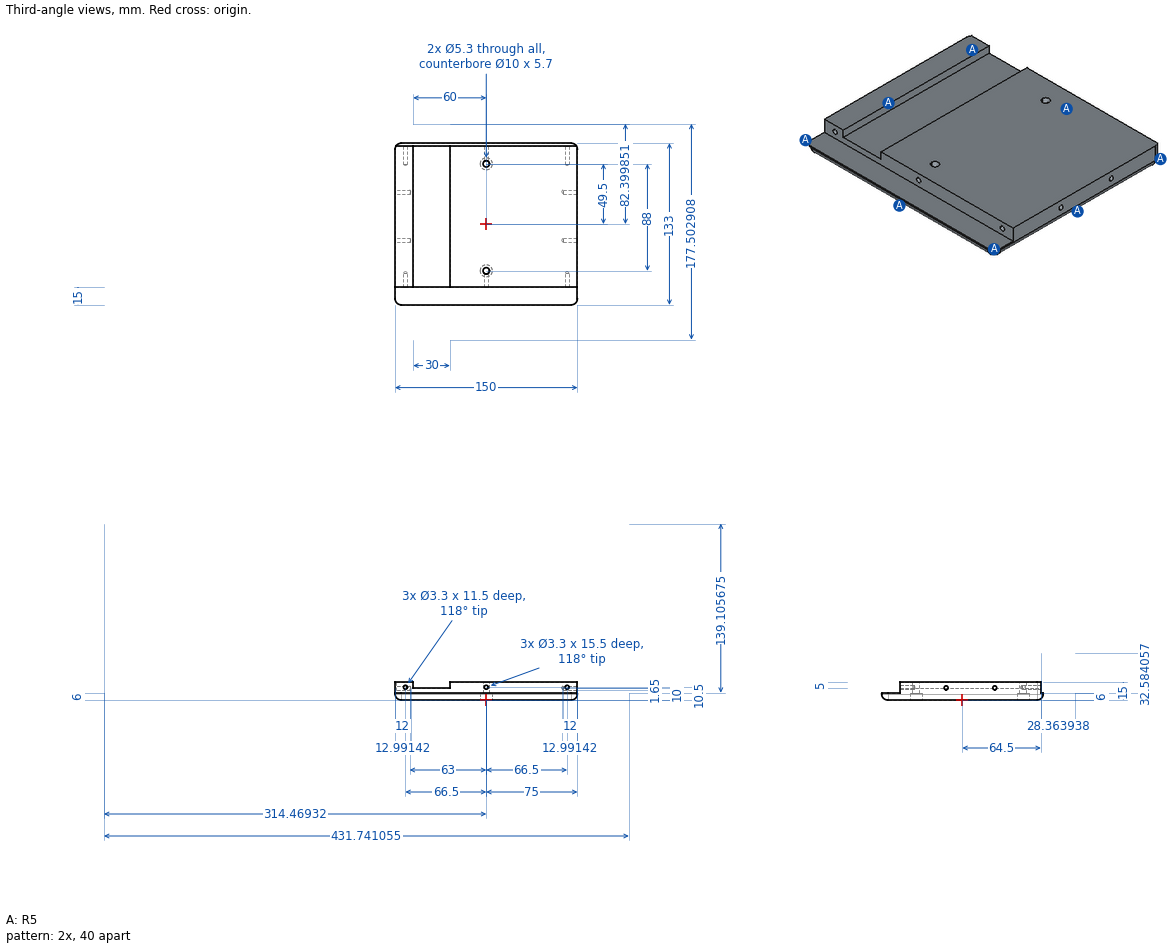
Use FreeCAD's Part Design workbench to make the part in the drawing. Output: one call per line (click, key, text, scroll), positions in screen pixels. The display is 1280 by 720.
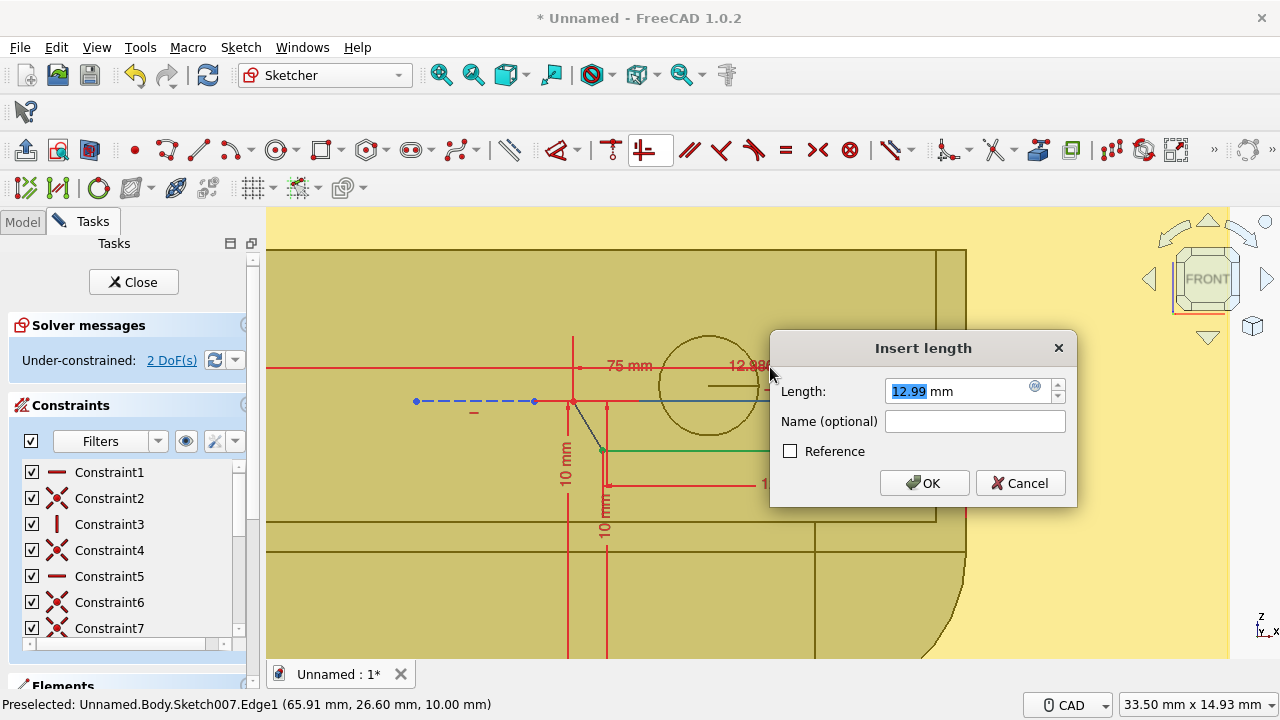
text(12.99142)
key(Return)
key(Escape)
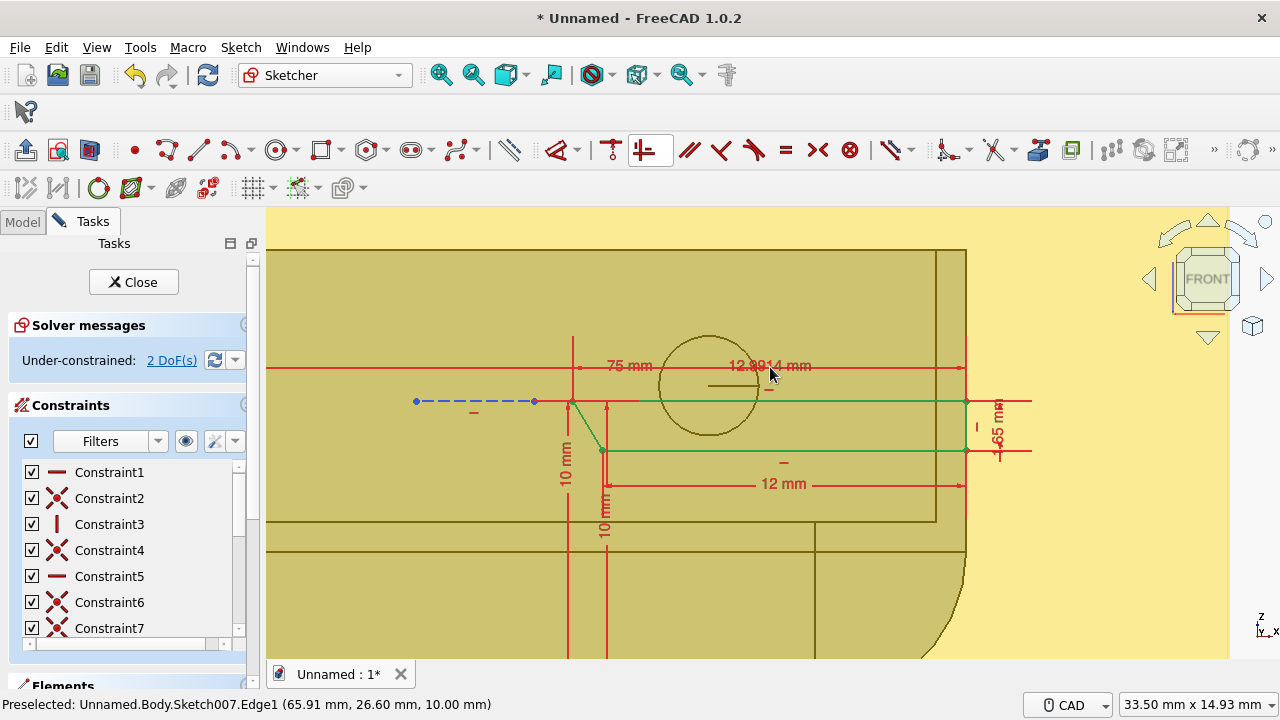
click(134, 282)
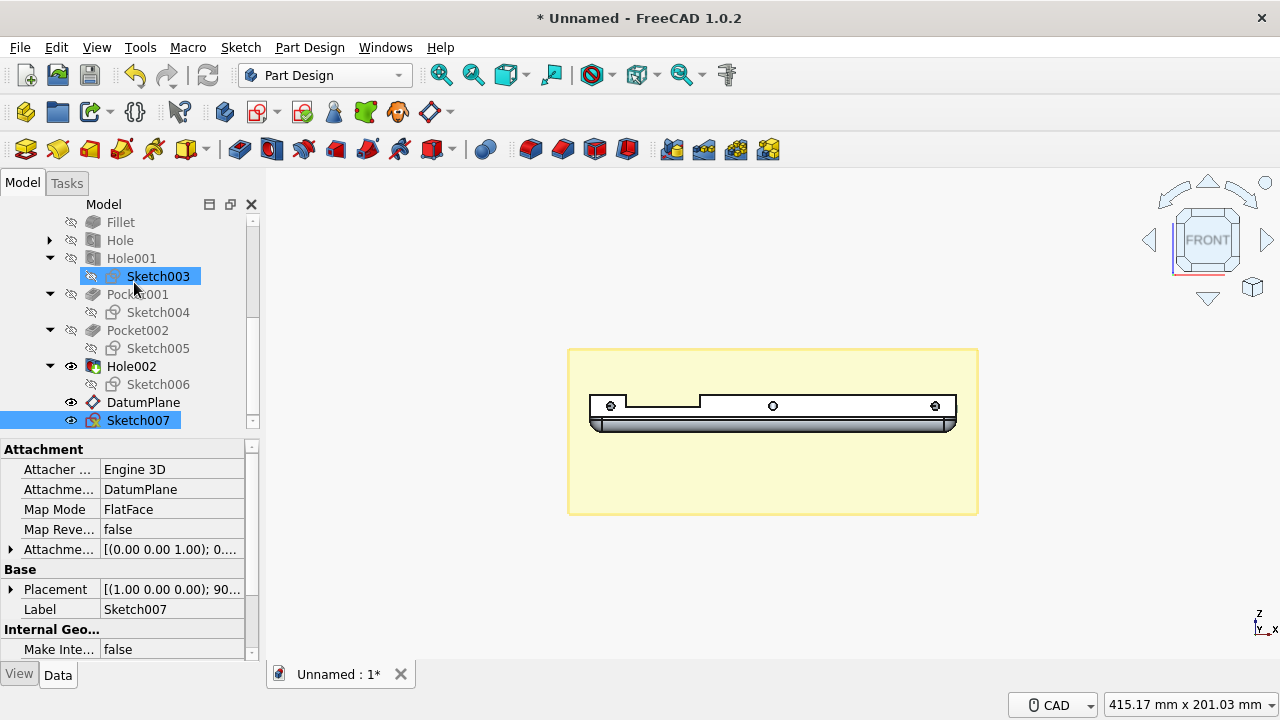
click(304, 150)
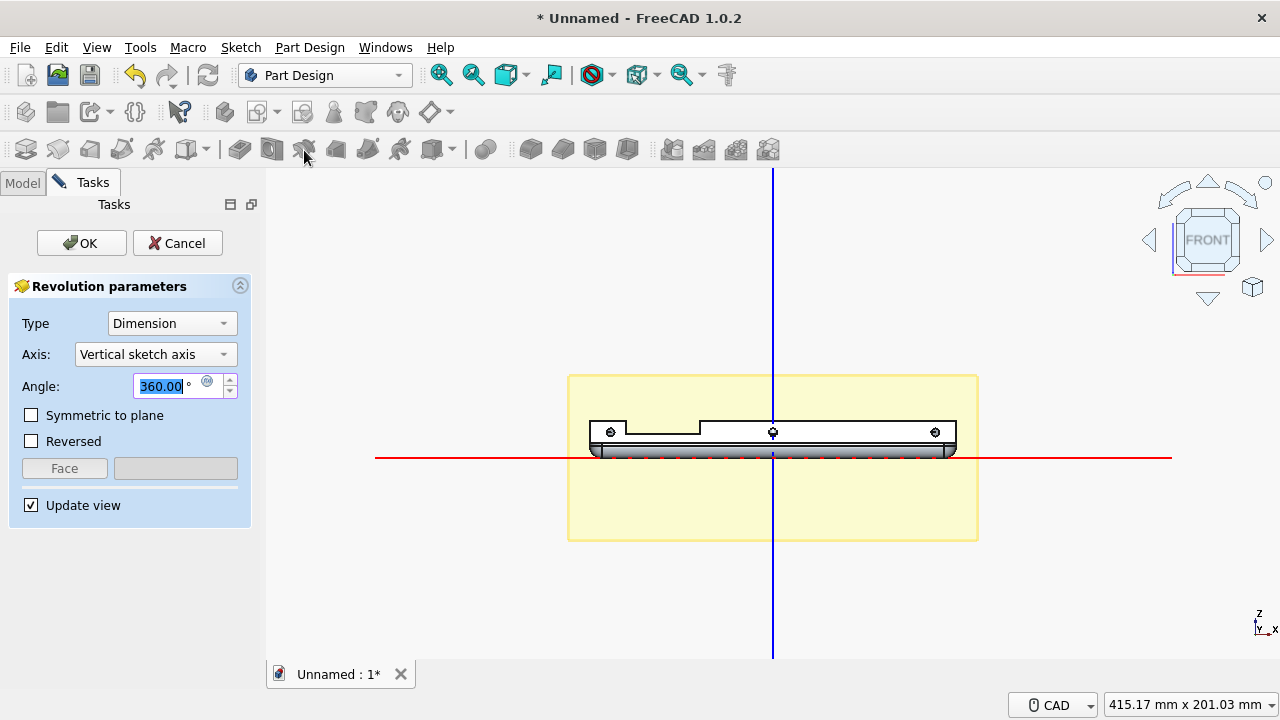
click(156, 354)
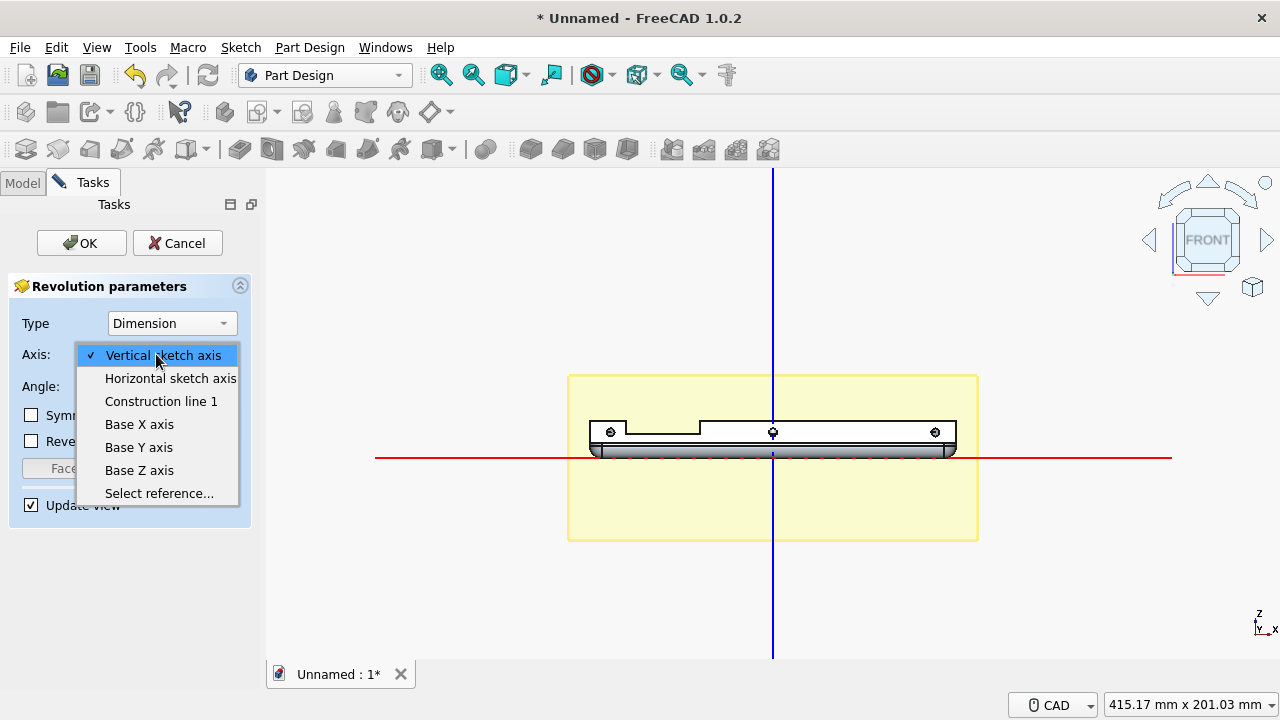
click(156, 402)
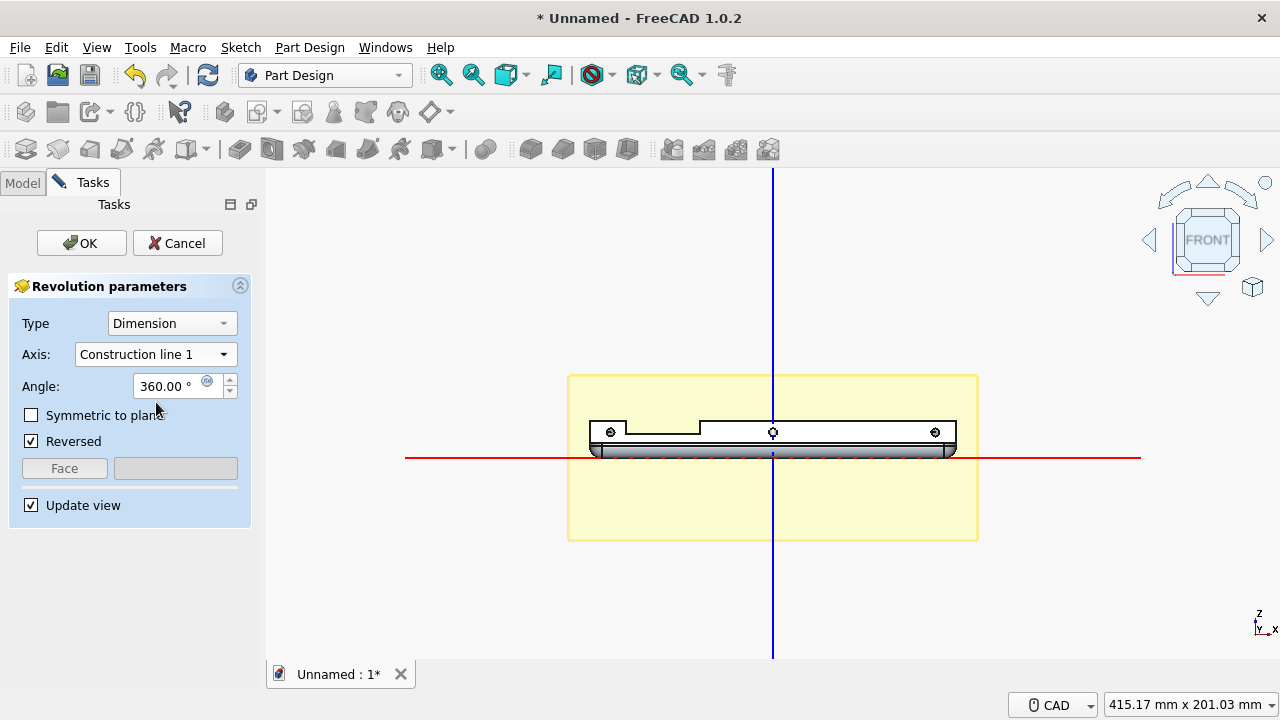
click(82, 243)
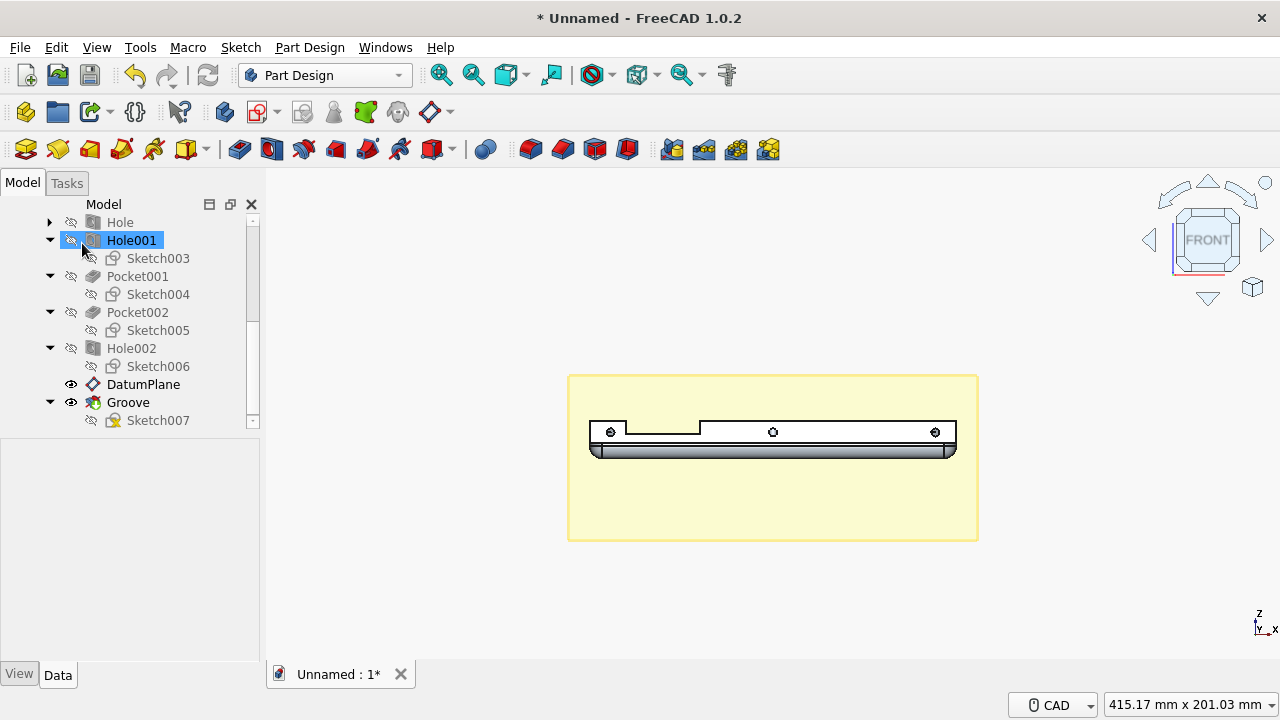
click(116, 384)
key(space)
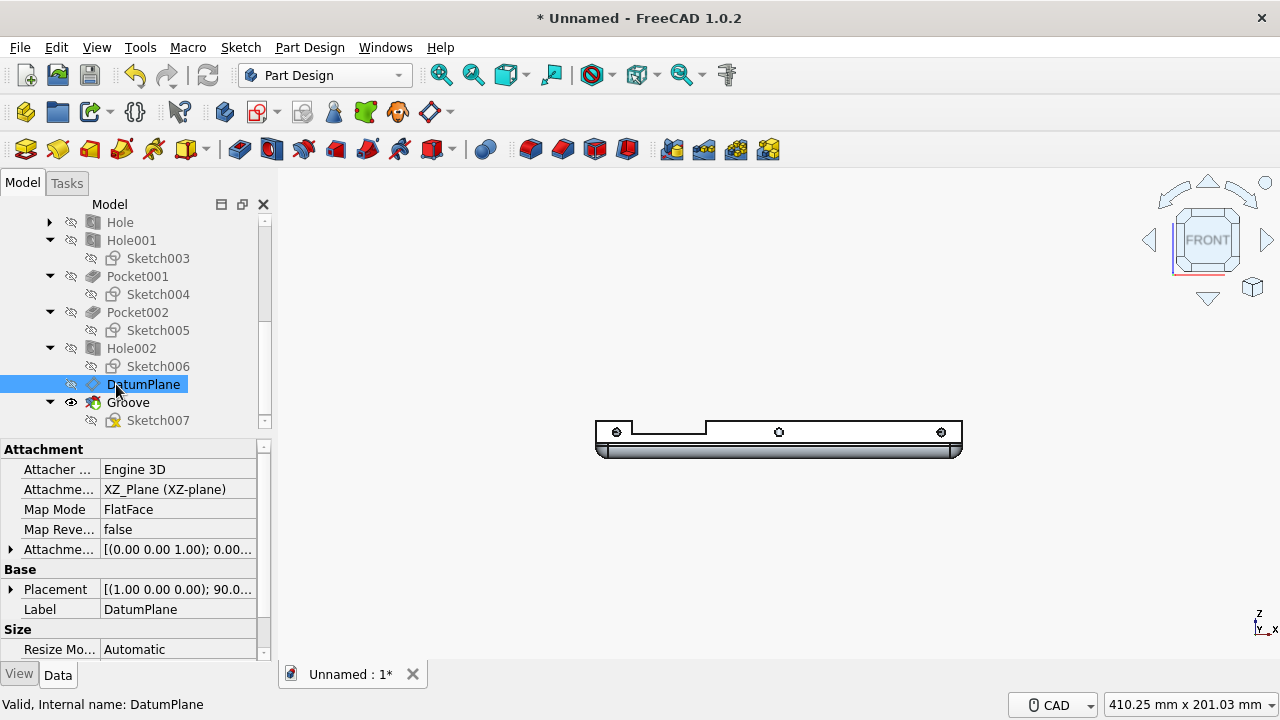
click(442, 76)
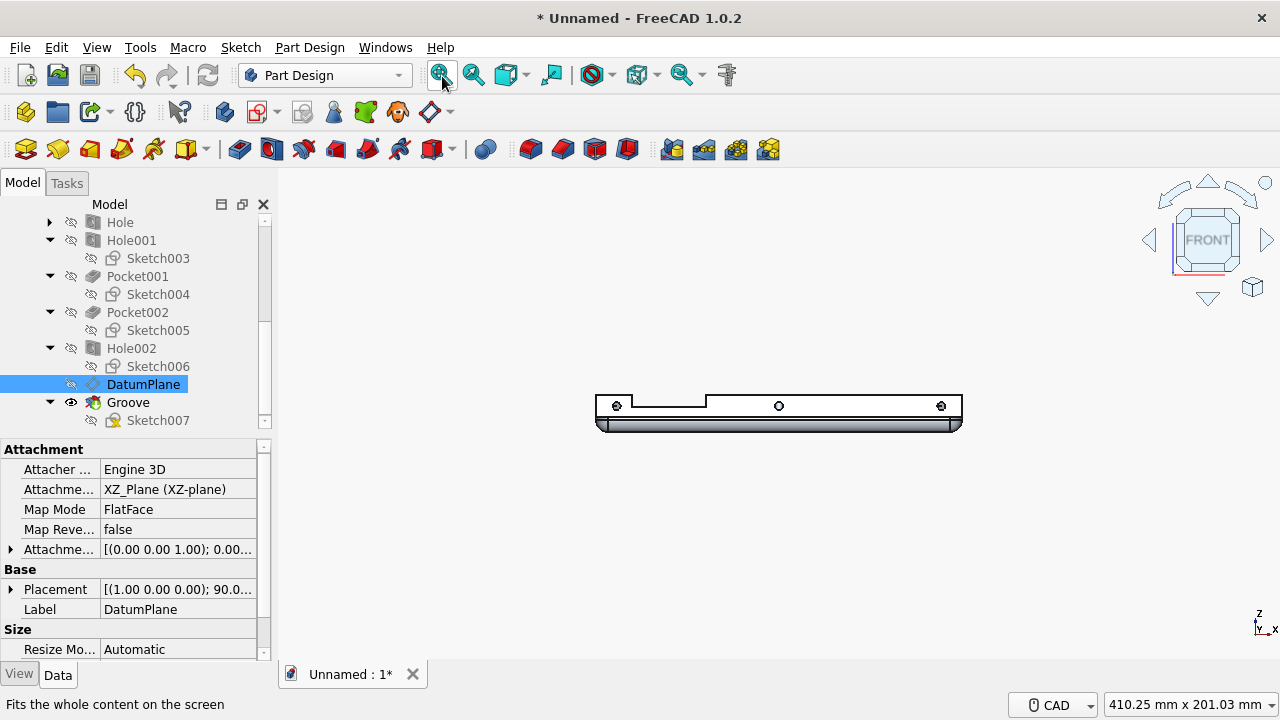
click(116, 402)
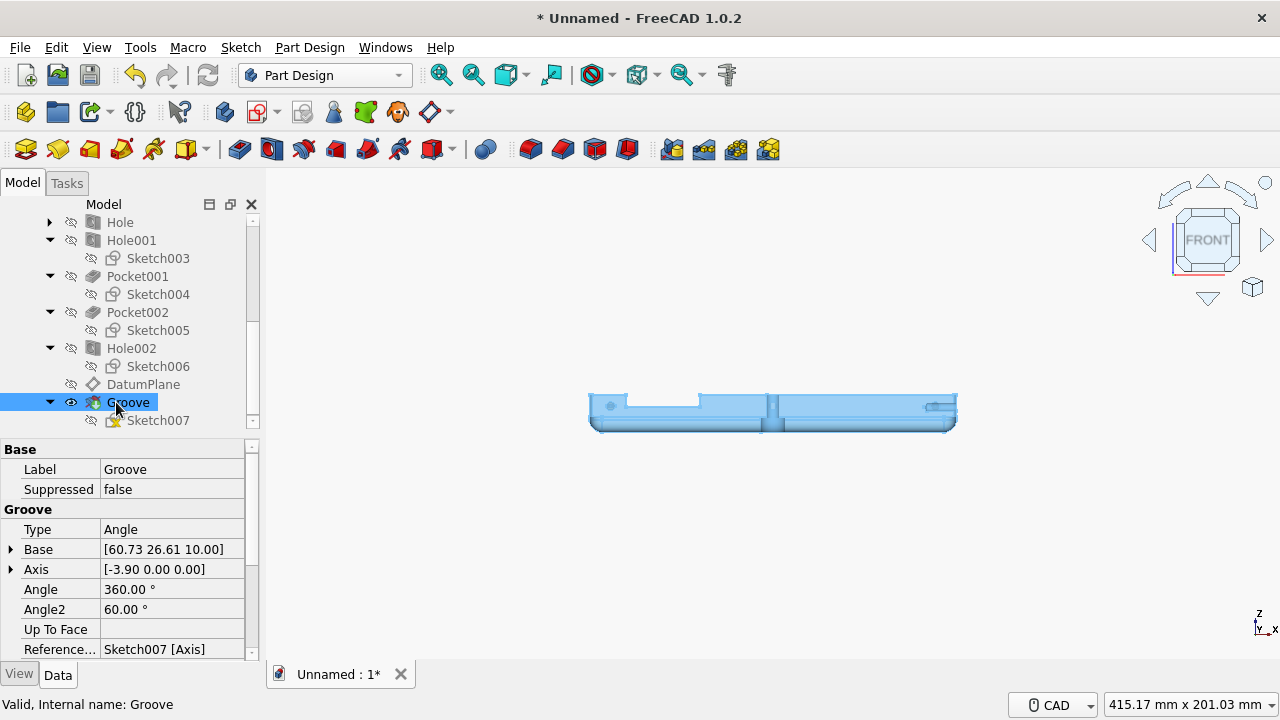
click(704, 150)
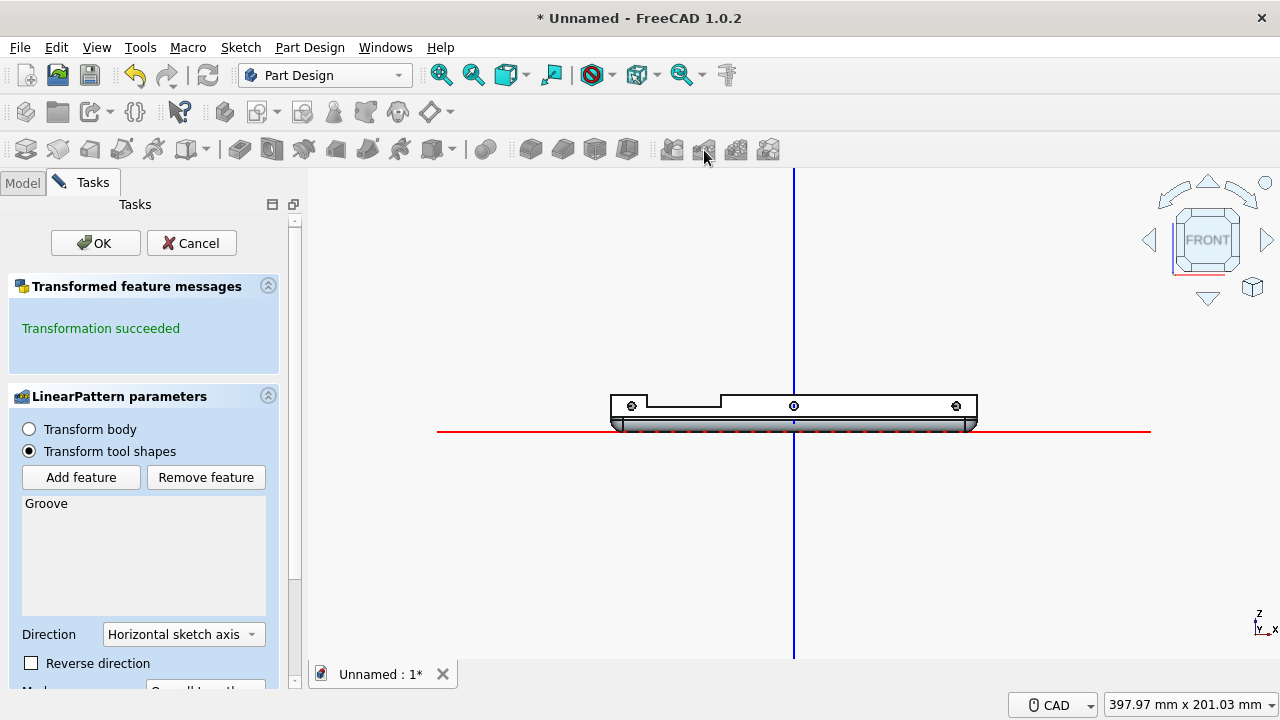
click(184, 634)